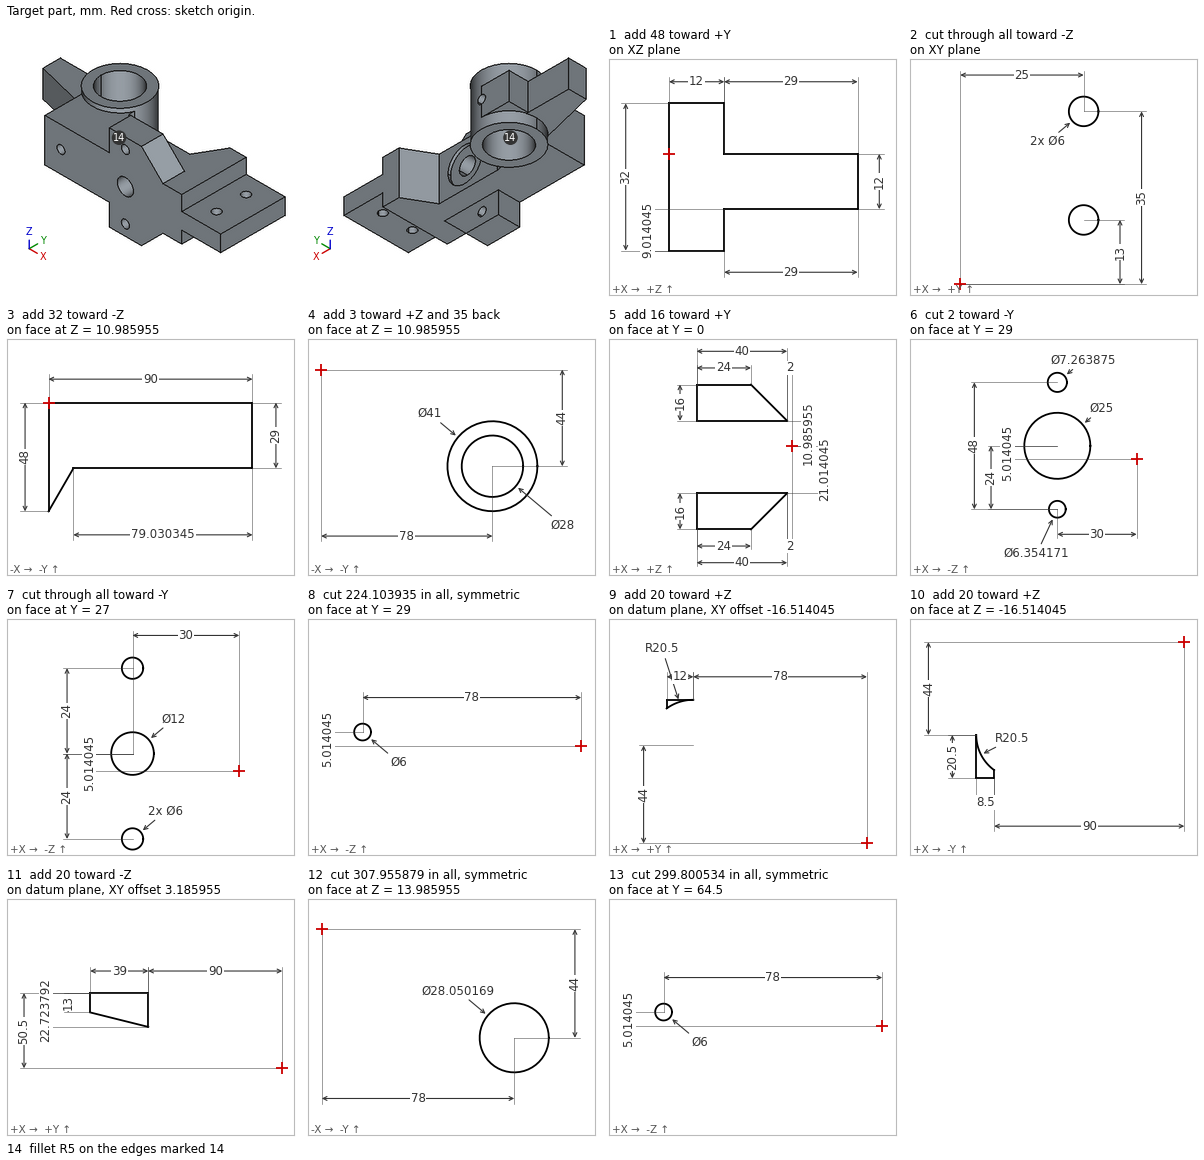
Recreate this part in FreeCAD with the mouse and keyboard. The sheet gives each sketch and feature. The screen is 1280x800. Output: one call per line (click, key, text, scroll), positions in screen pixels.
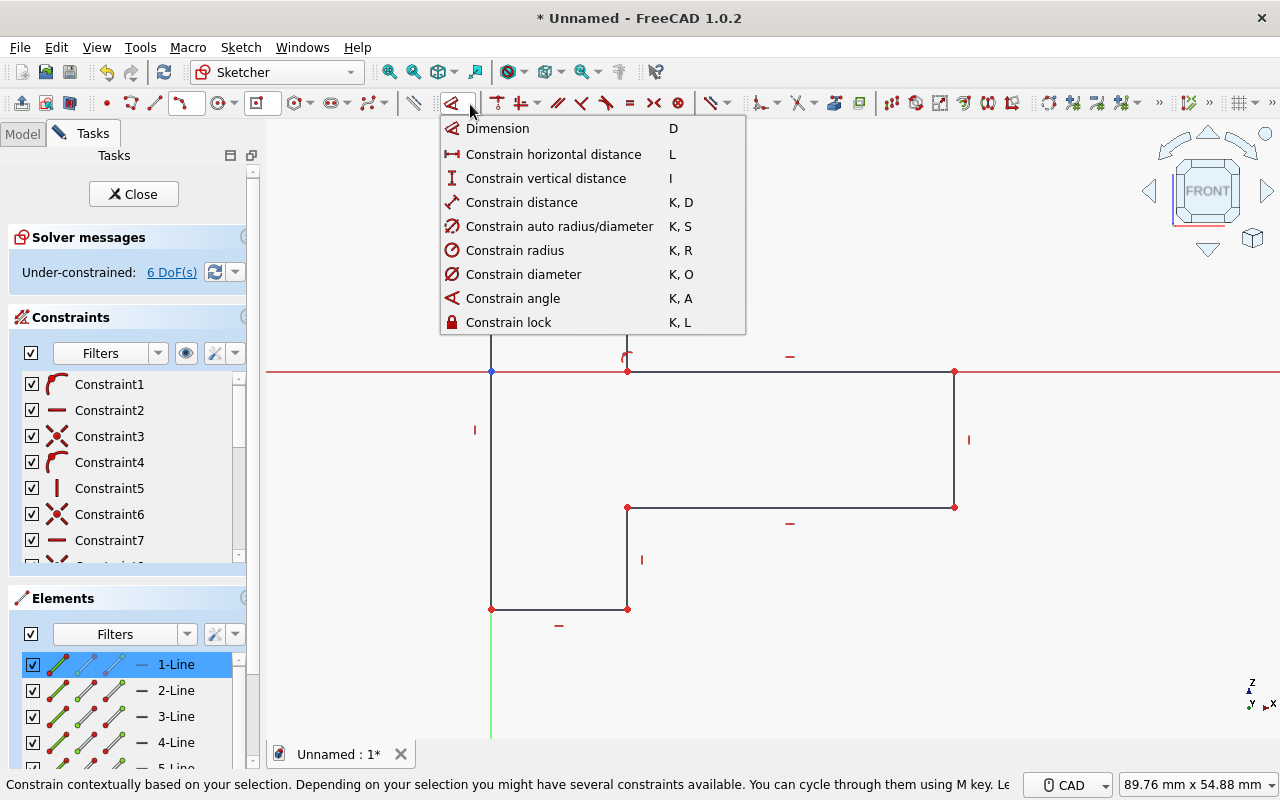
click(593, 154)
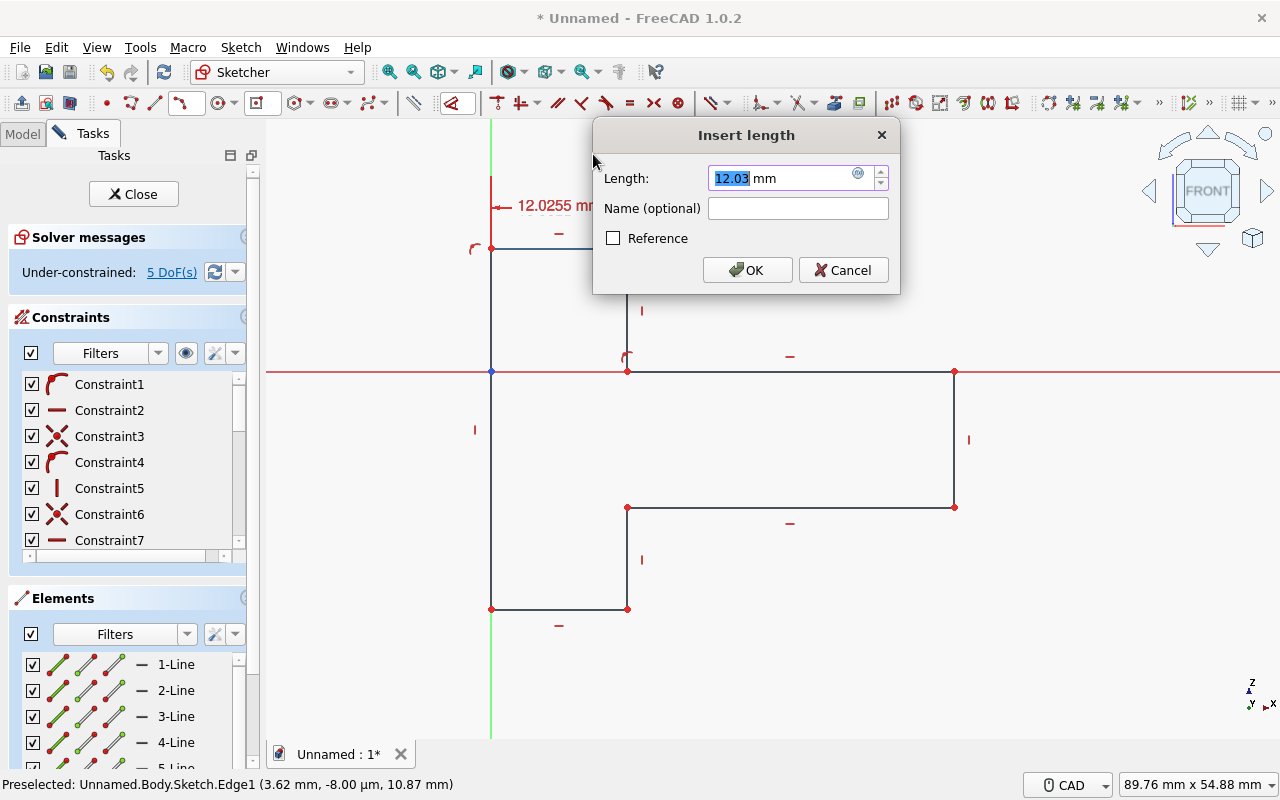
text(12)
key(Return)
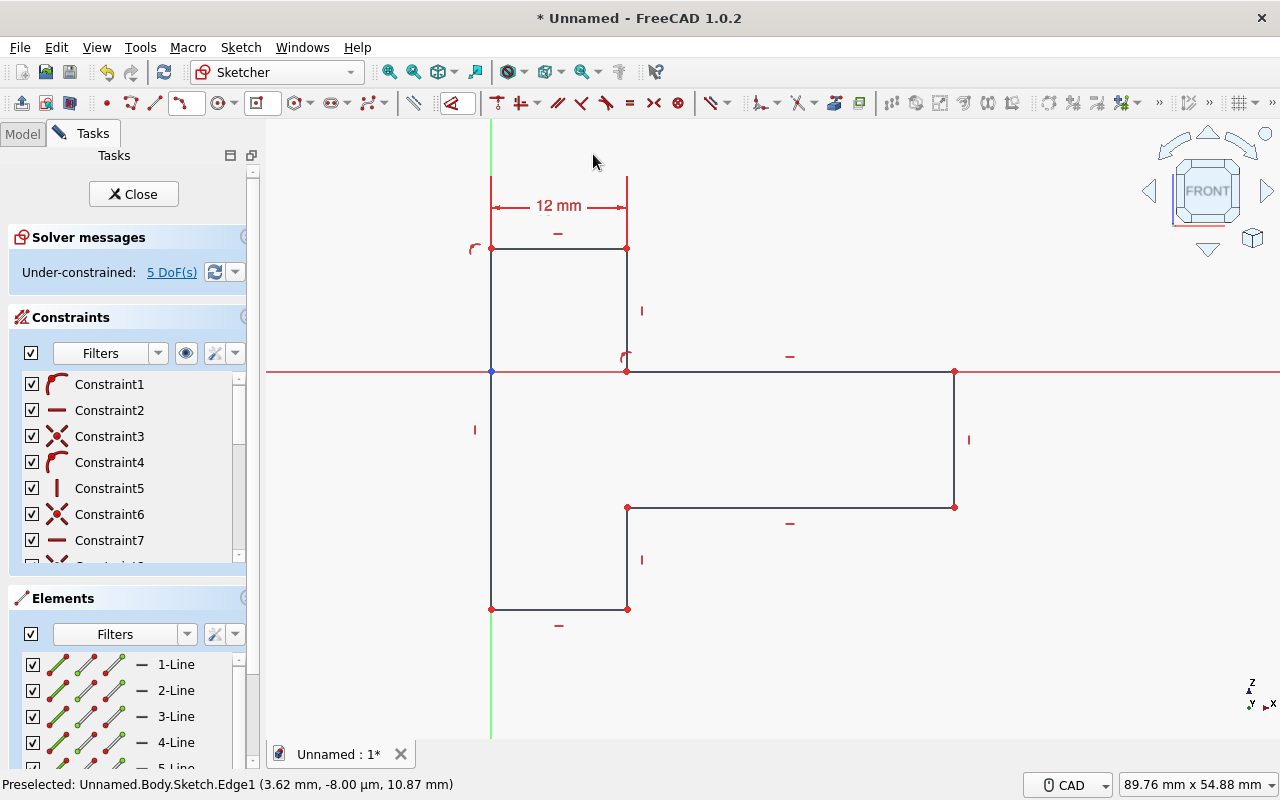
click(725, 372)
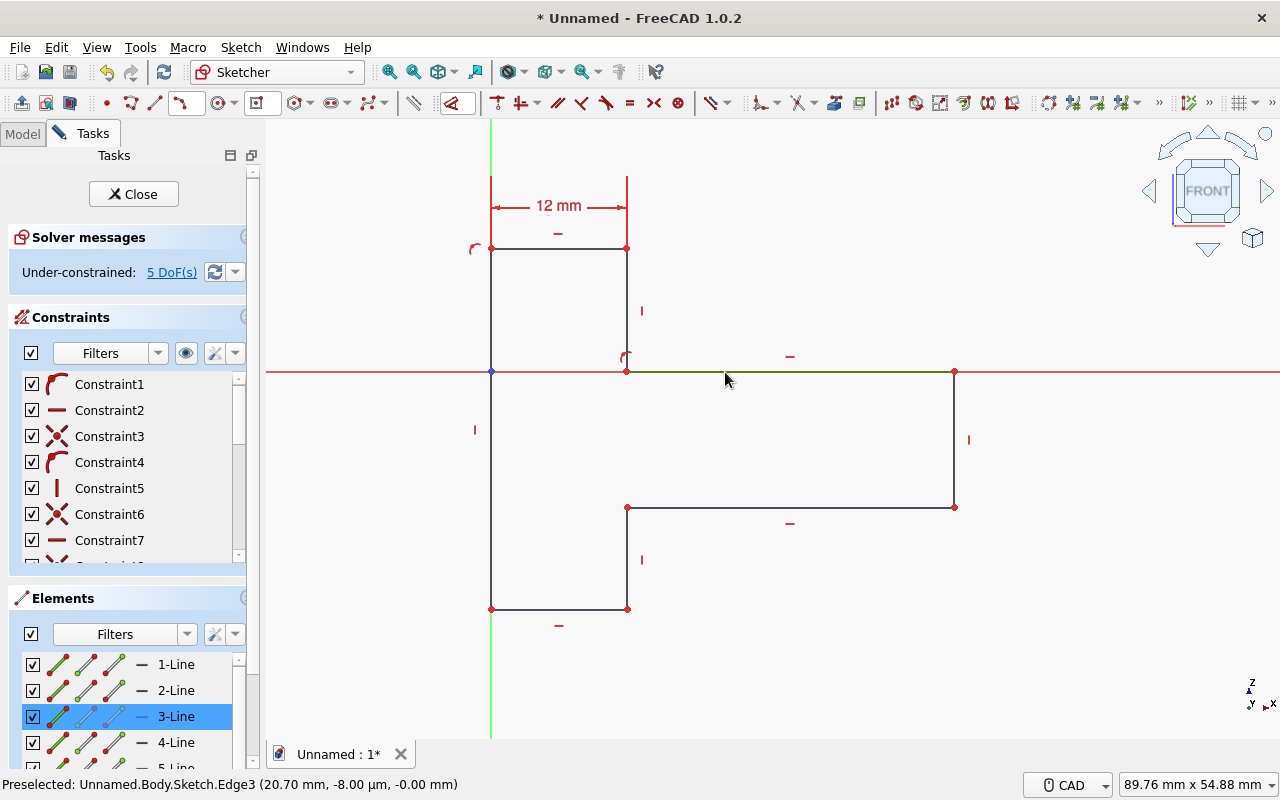
key(l)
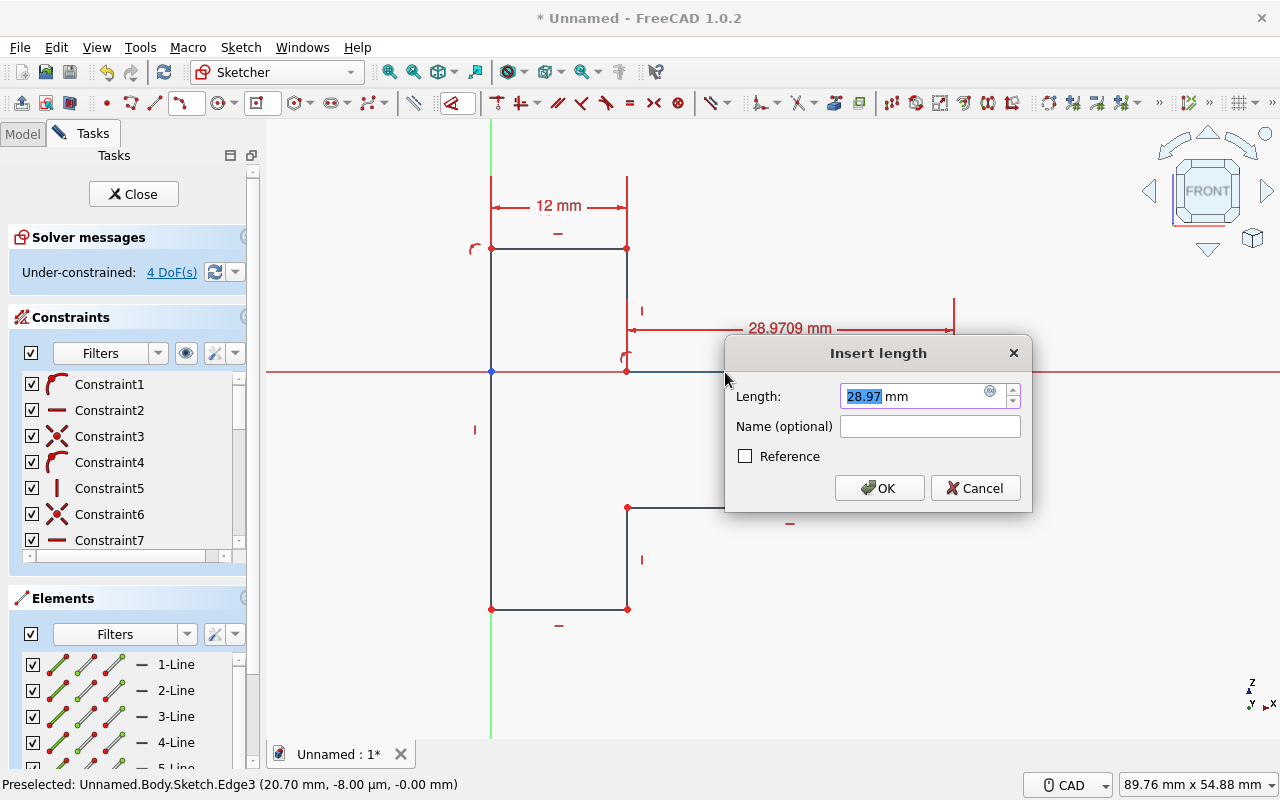
text(29)
key(Return)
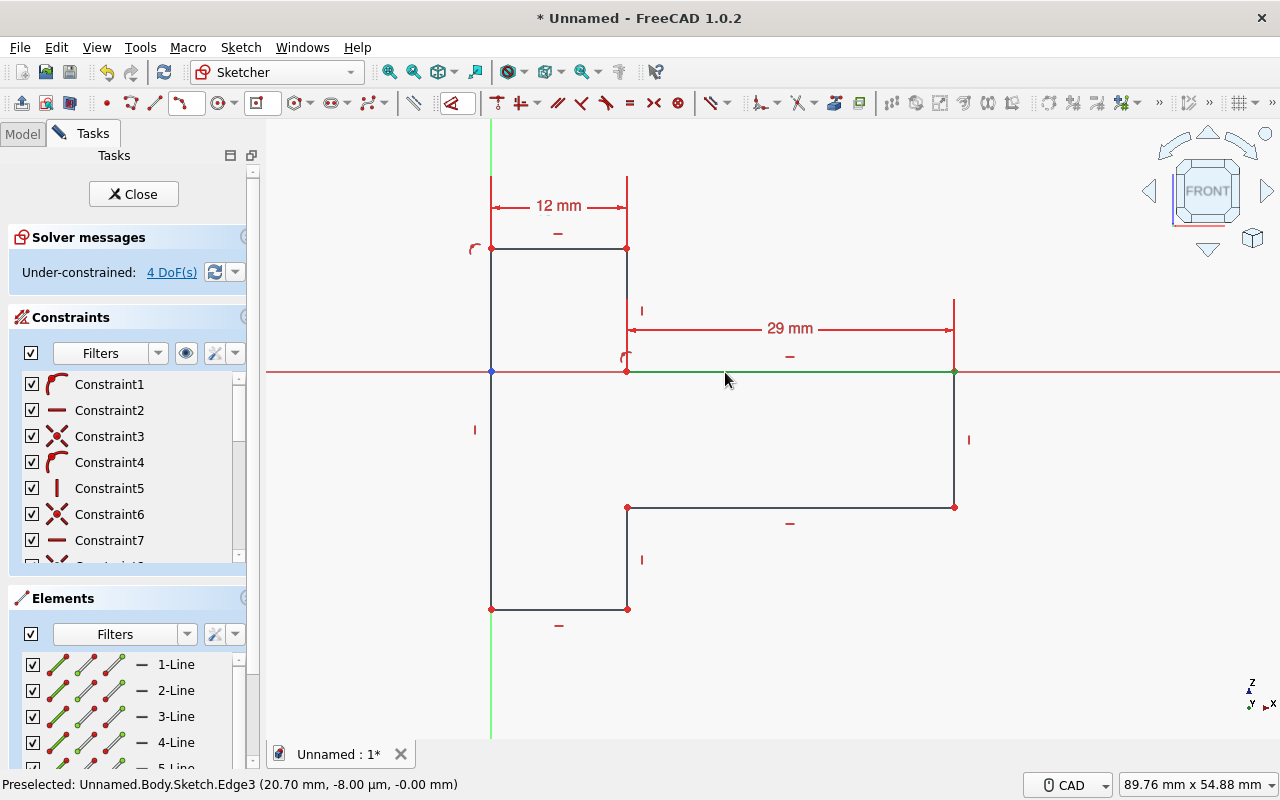
click(954, 413)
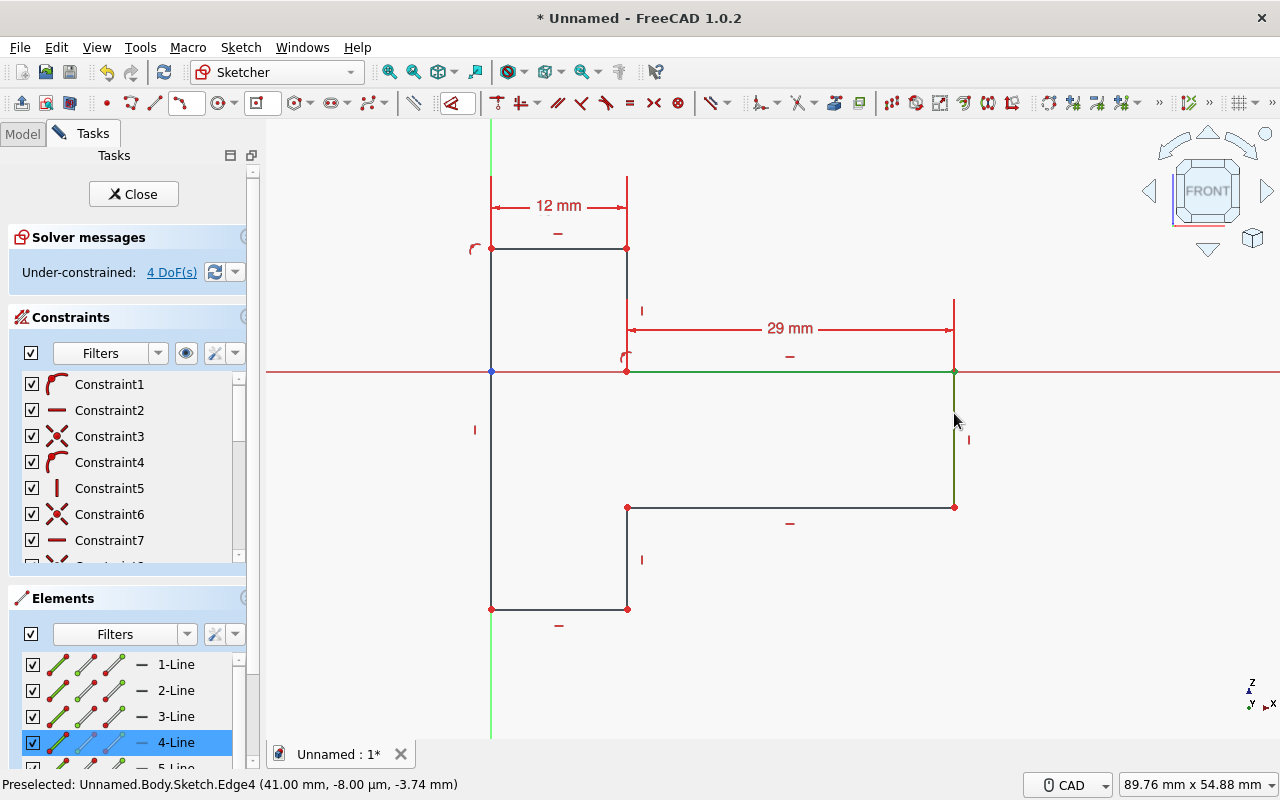
key(i)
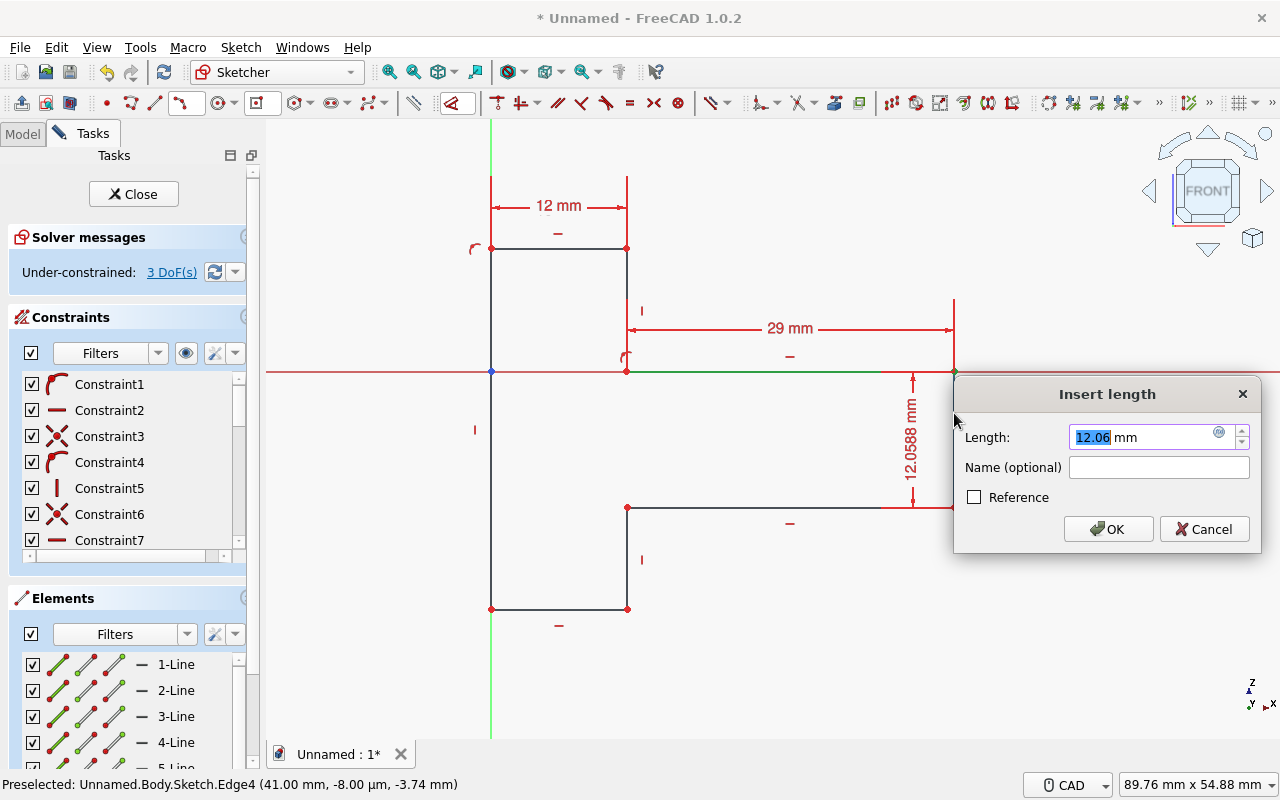
text(12)
key(Return)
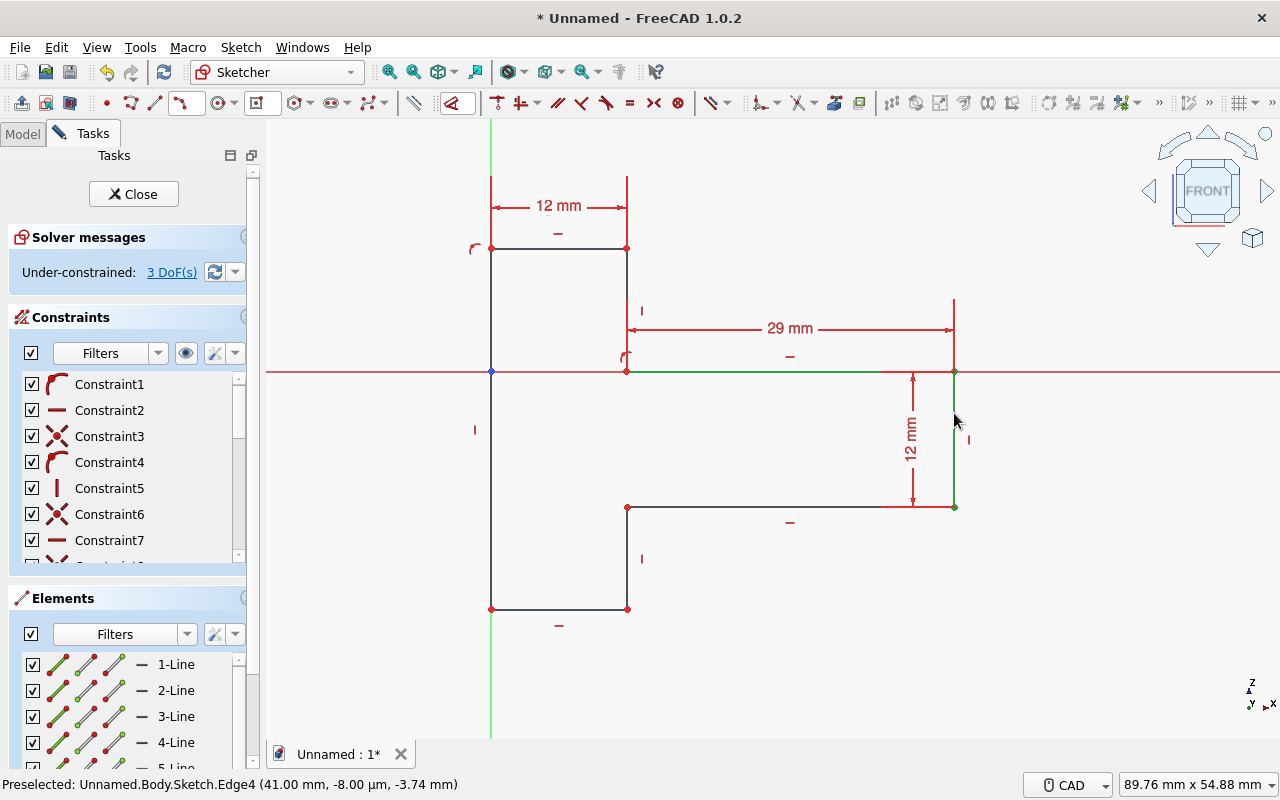
click(856, 507)